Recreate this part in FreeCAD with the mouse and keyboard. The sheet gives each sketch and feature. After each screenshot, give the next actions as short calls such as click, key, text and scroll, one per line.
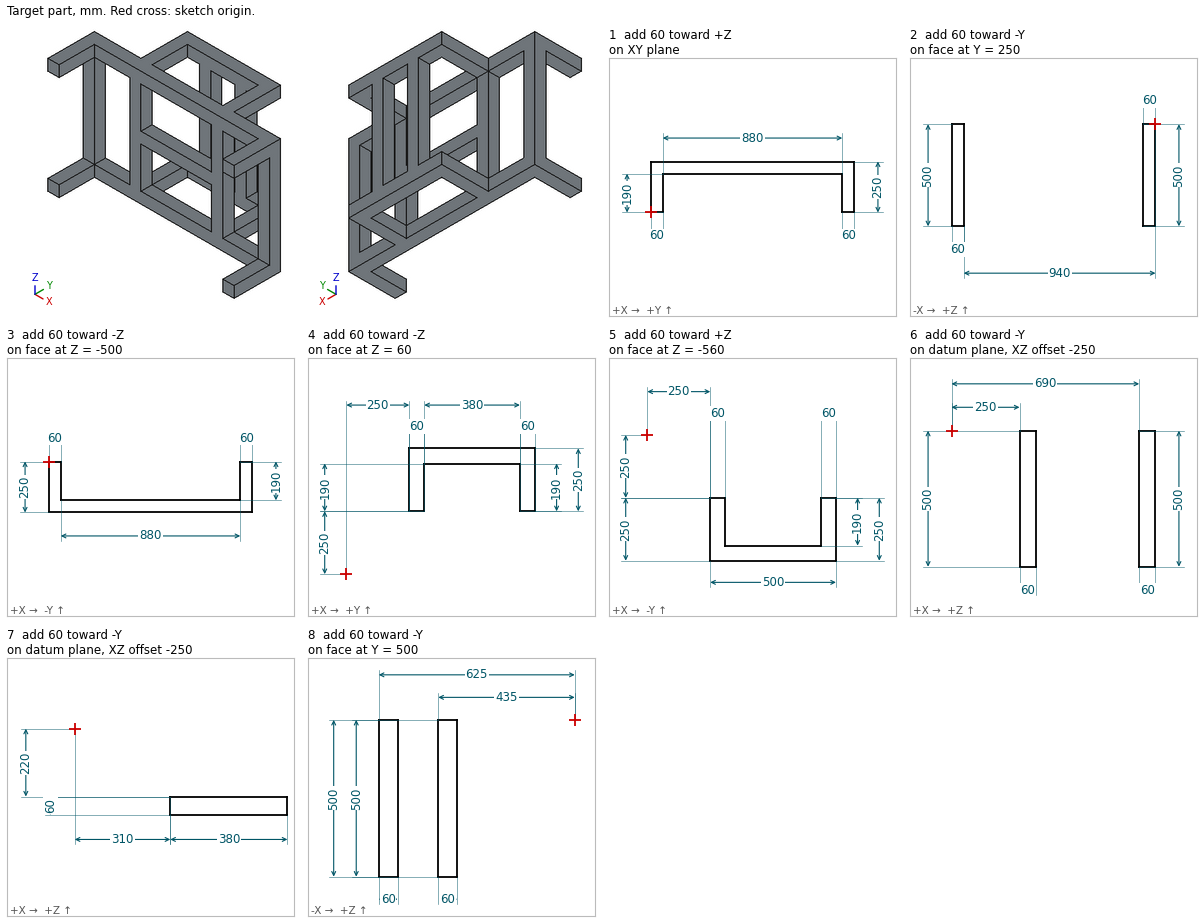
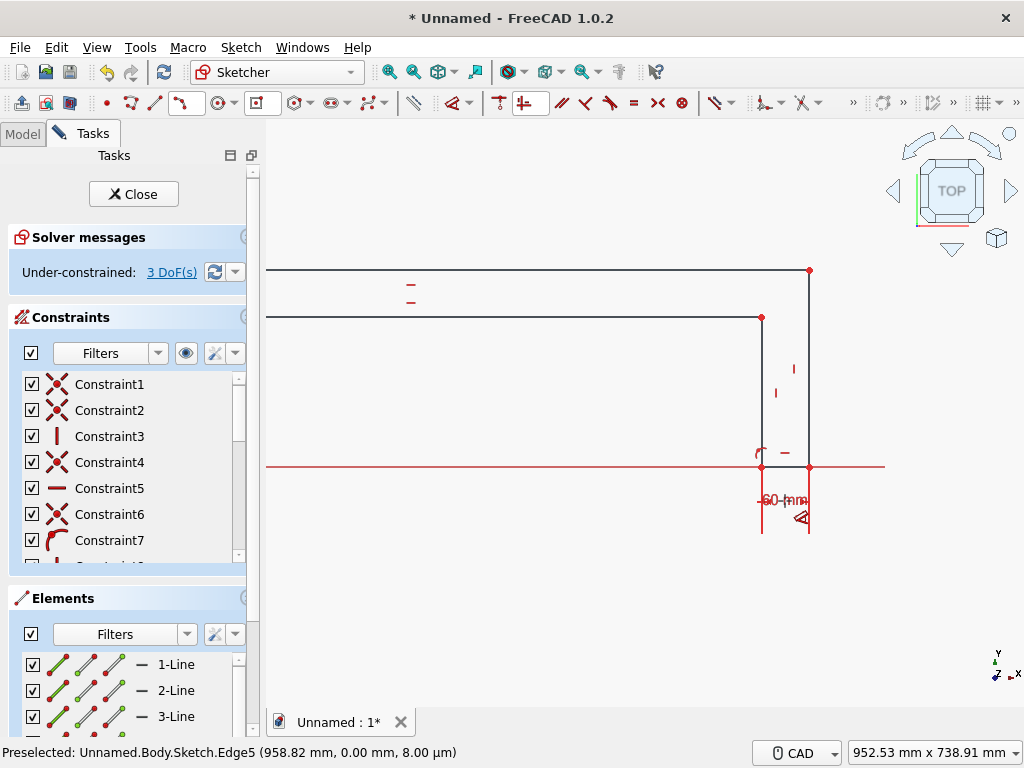
scroll(778, 468, down, 3)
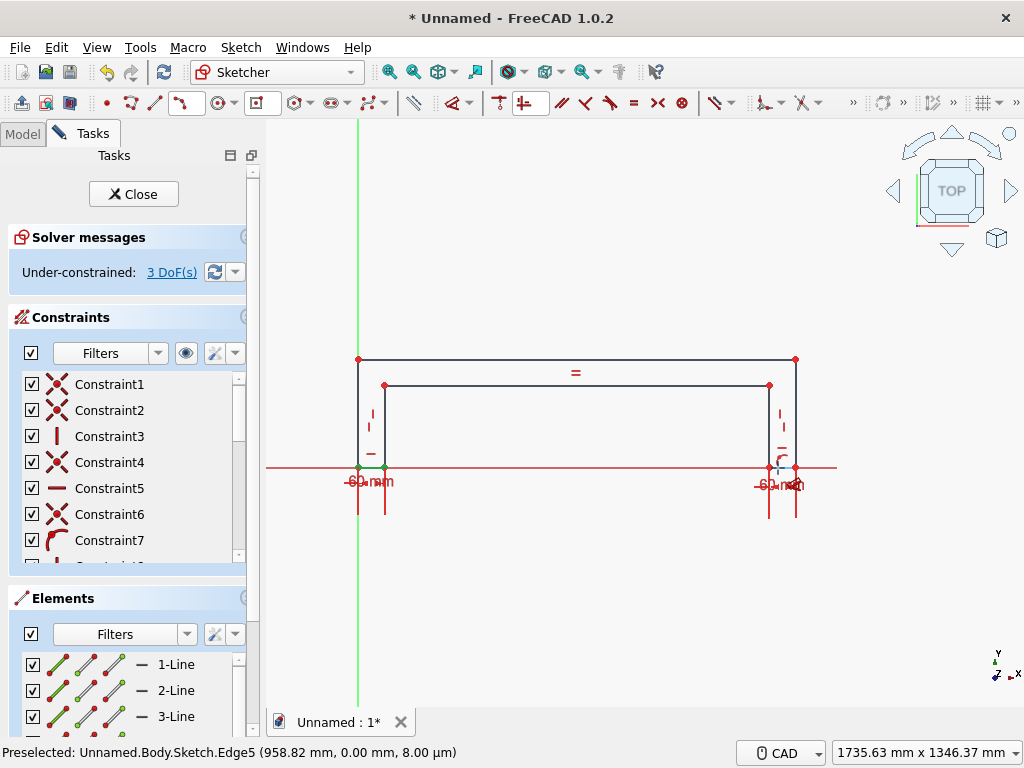
click(385, 443)
click(419, 427)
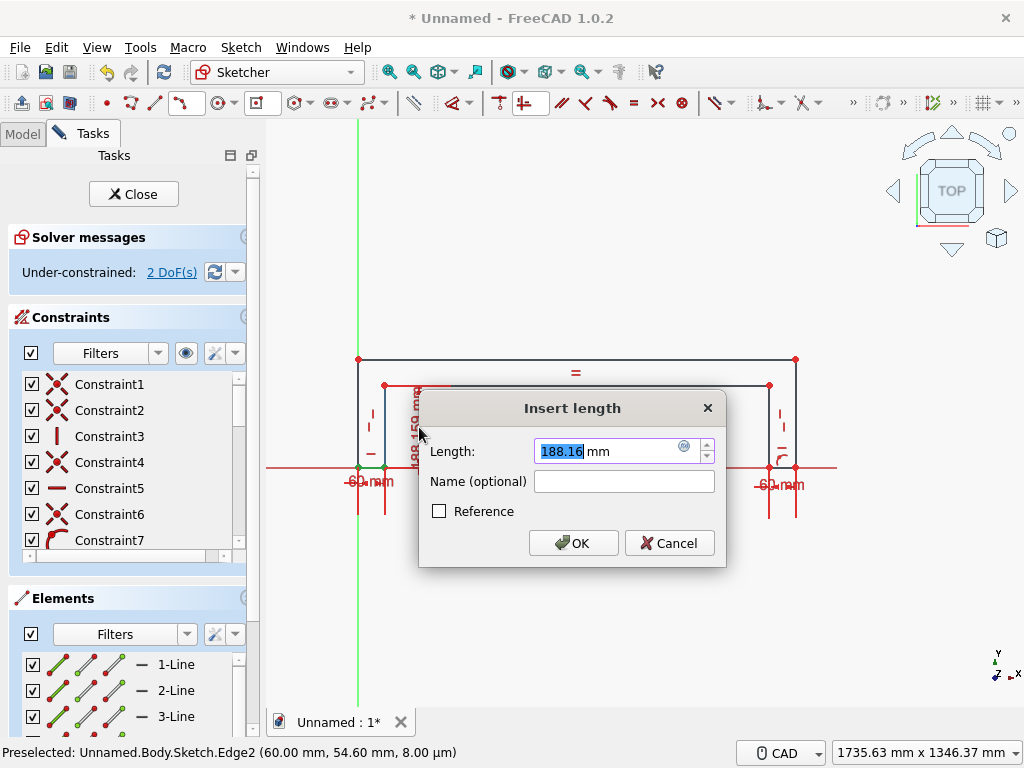
text(190)
key(Return)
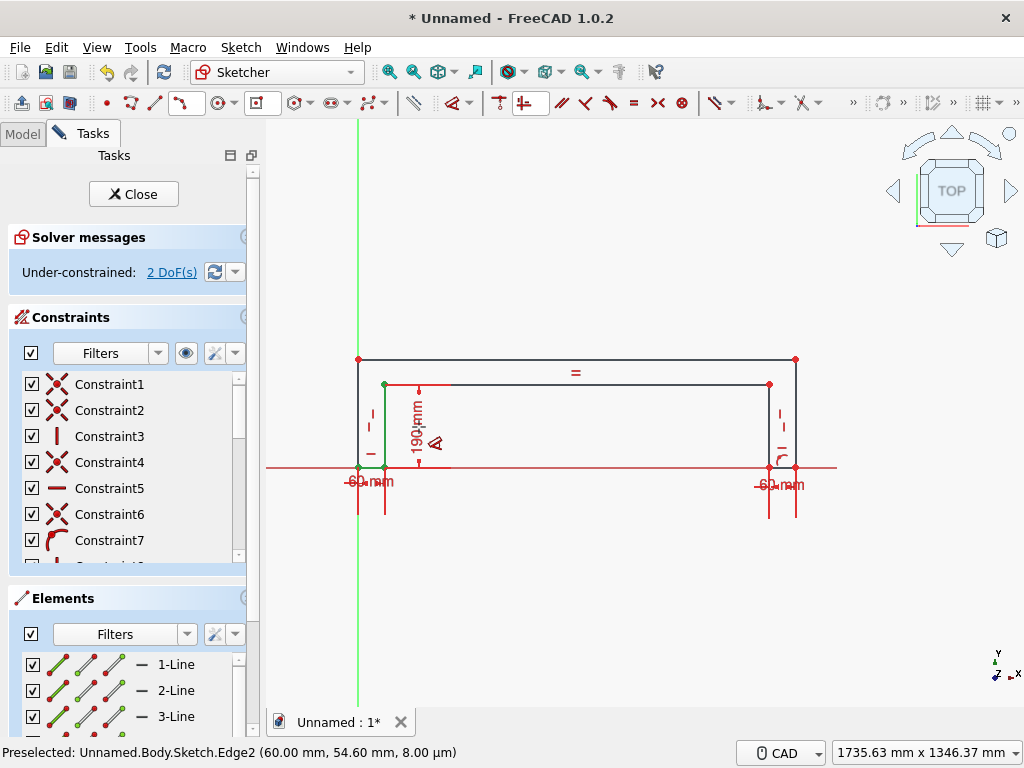
click(500, 385)
click(577, 419)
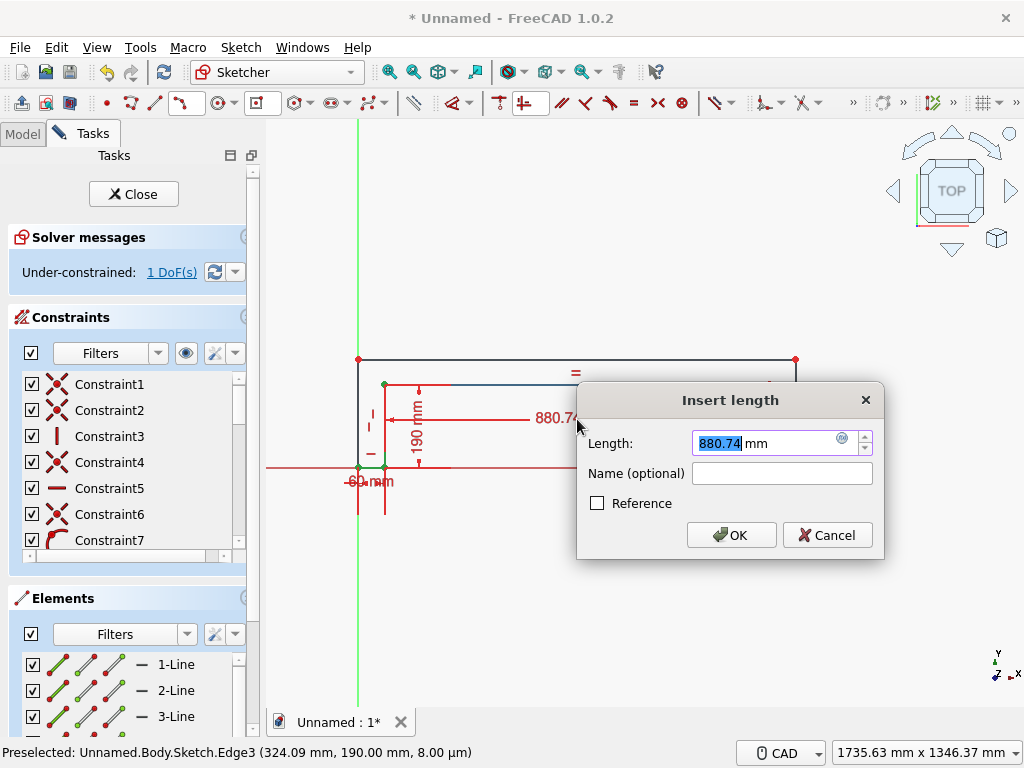
text(880)
key(Return)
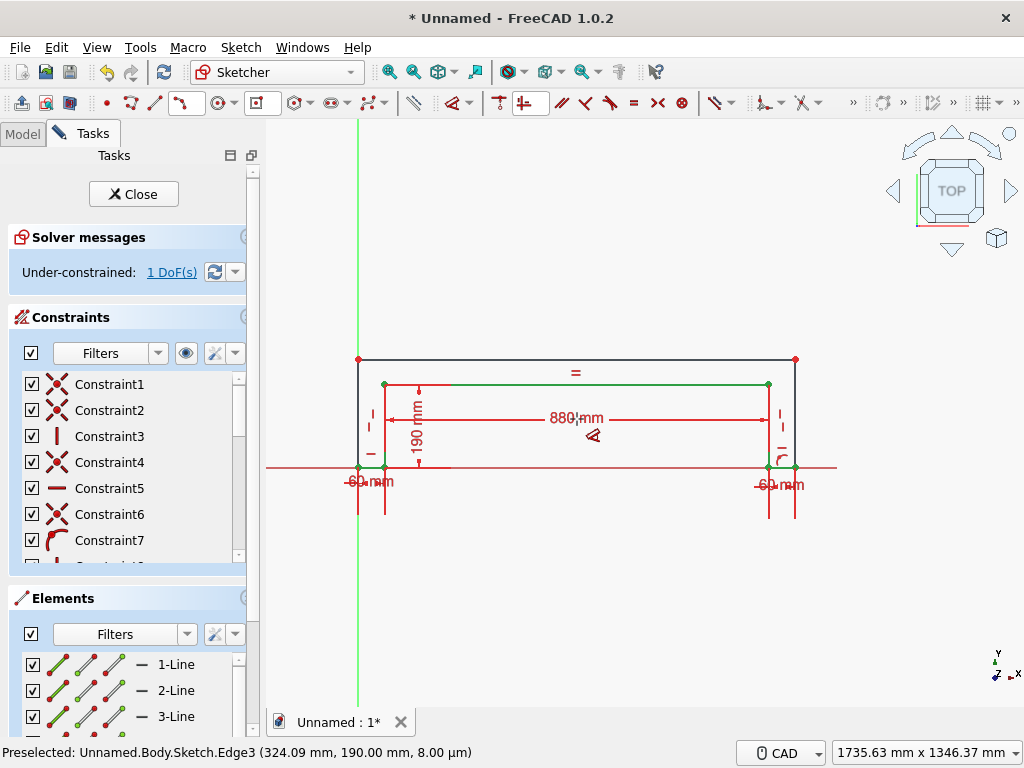
click(795, 435)
click(829, 414)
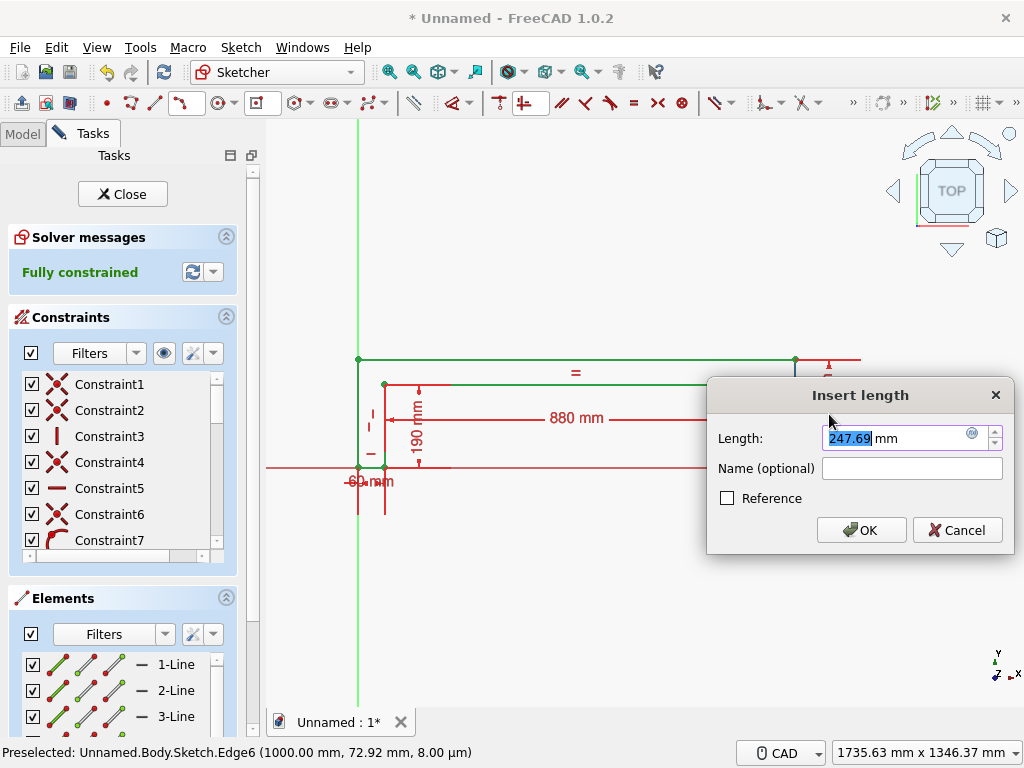
text(250)
key(Return)
key(Escape)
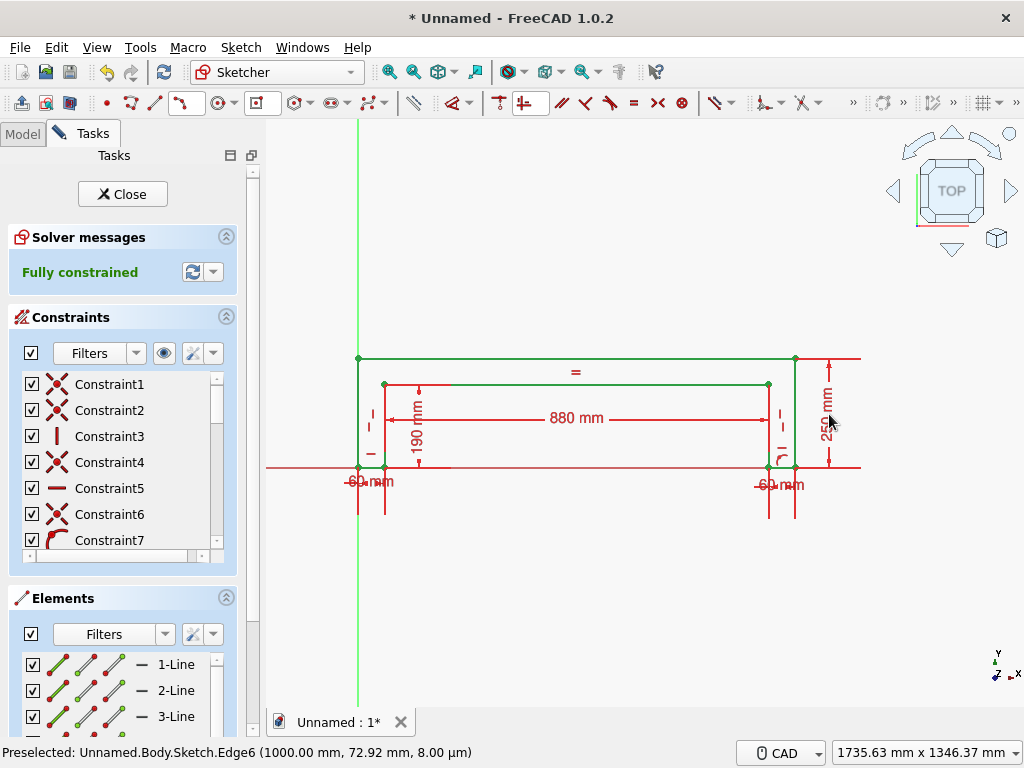
click(123, 194)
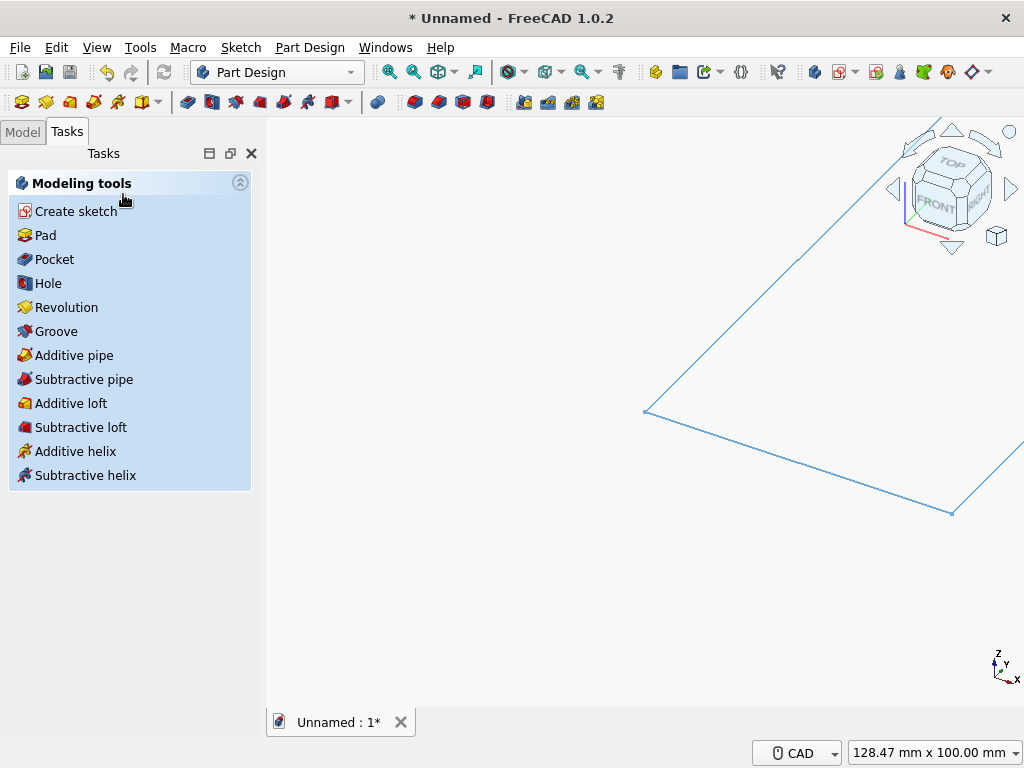
click(22, 102)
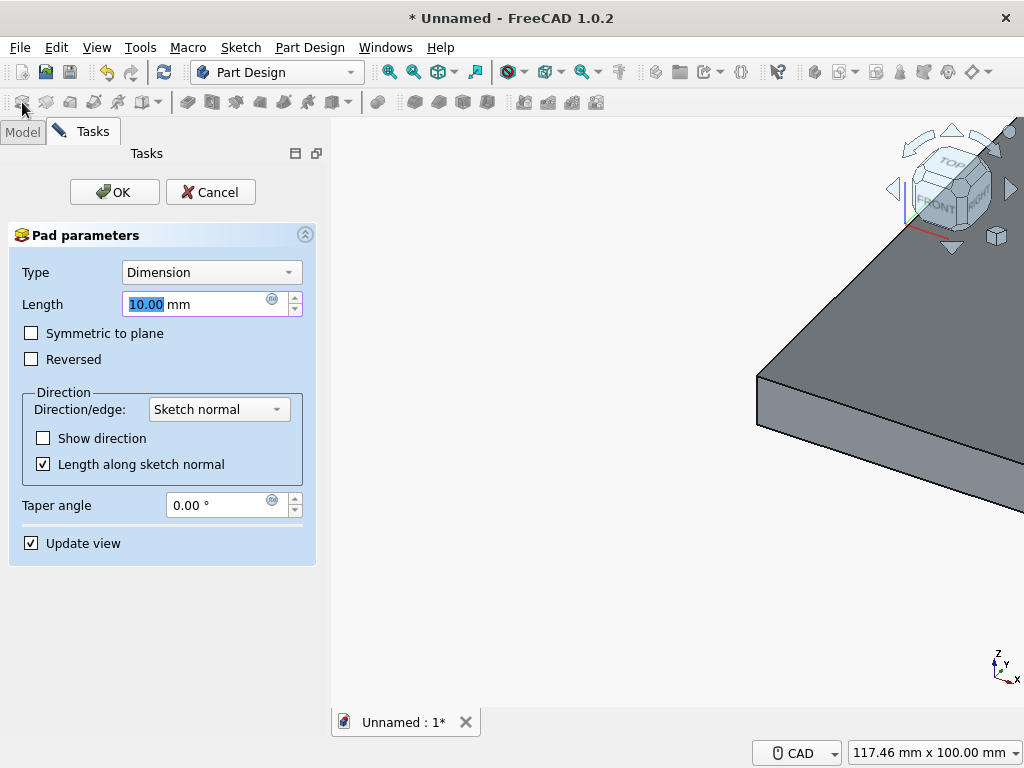
text(60)
key(Tab)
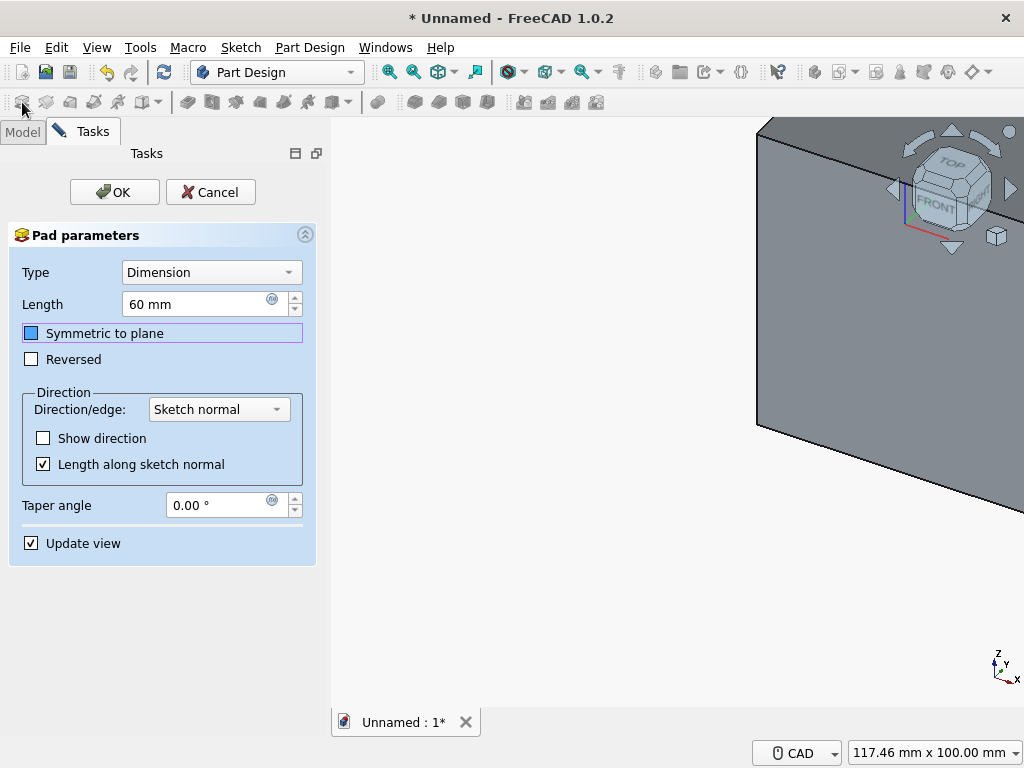
click(115, 192)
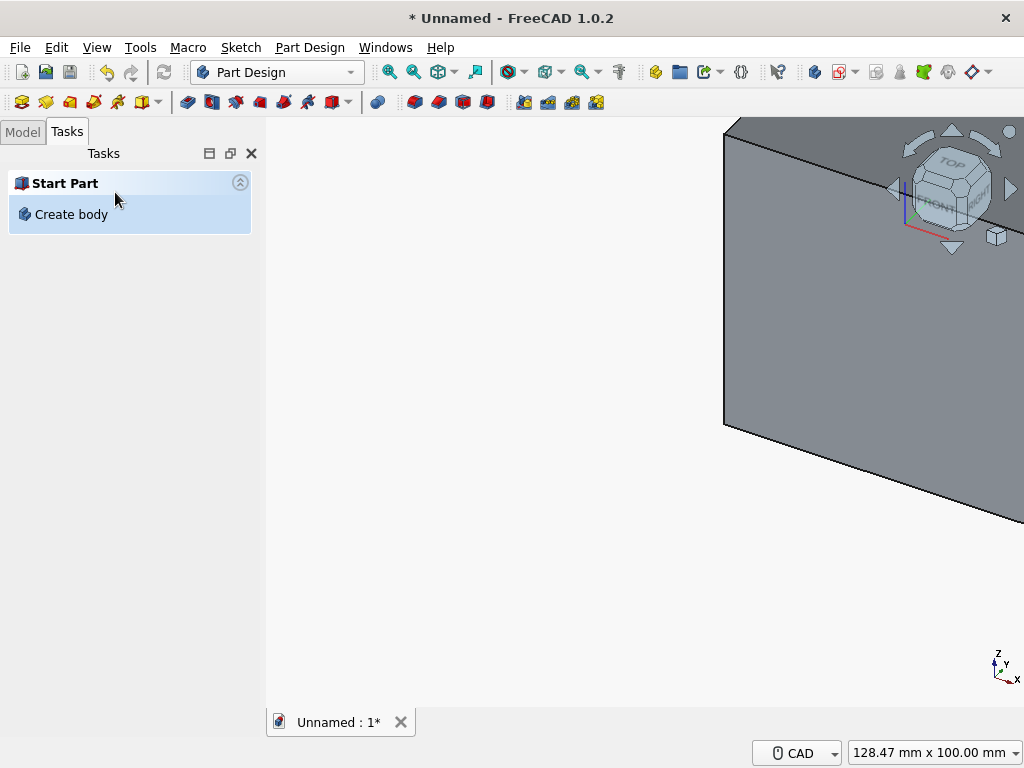
click(390, 72)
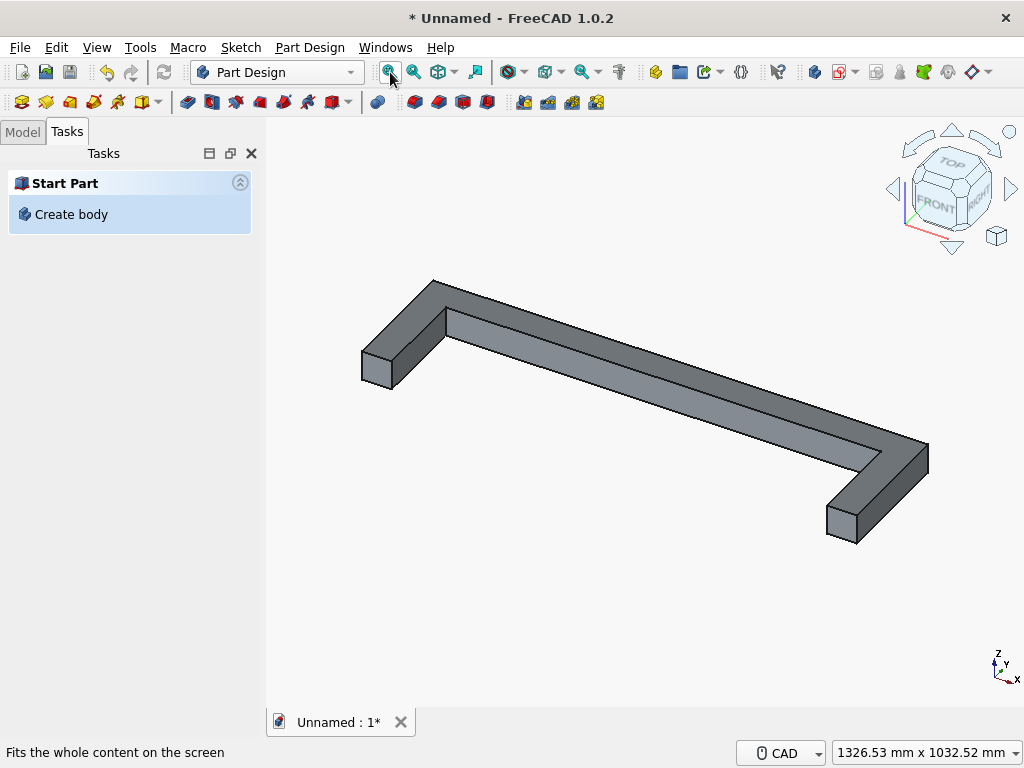
key(4)